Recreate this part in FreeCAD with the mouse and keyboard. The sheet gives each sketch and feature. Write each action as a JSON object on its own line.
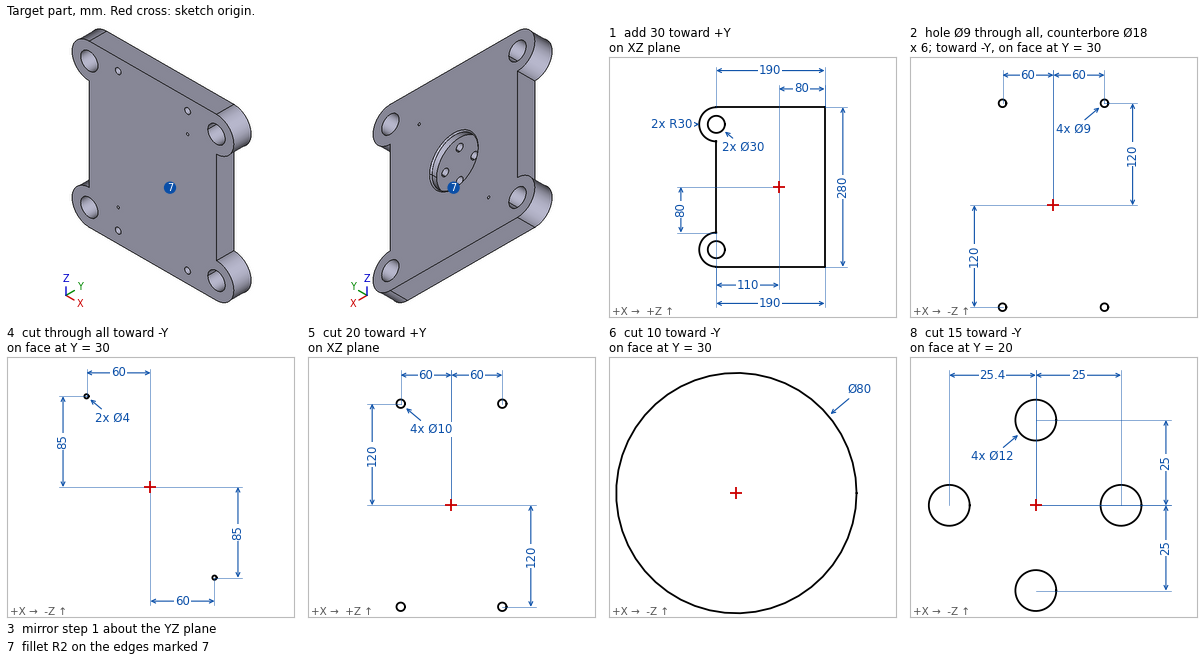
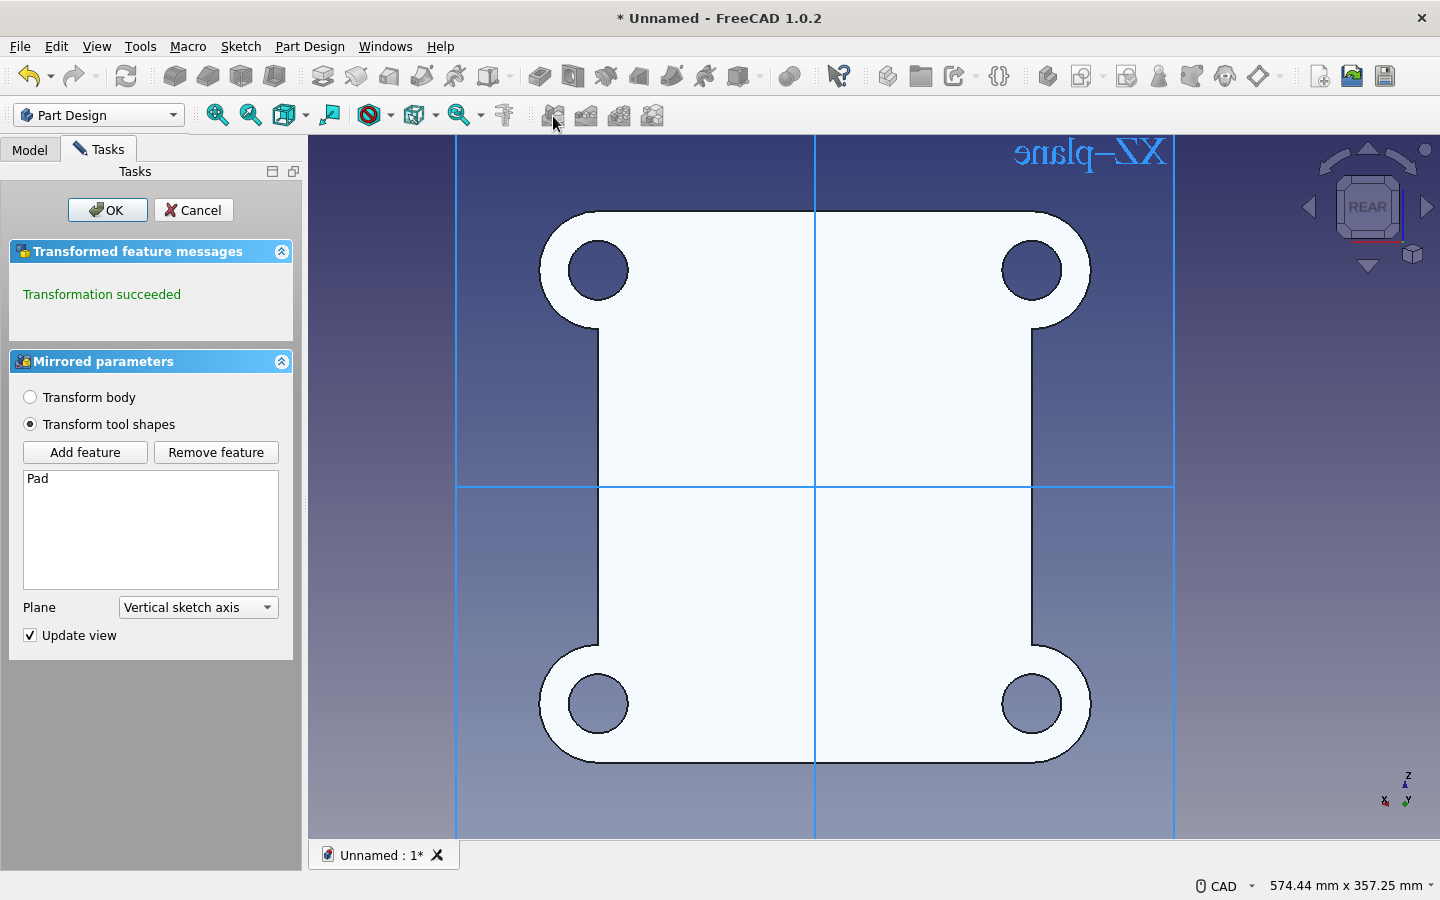
{"action": "left_click", "coordinate": [199, 608]}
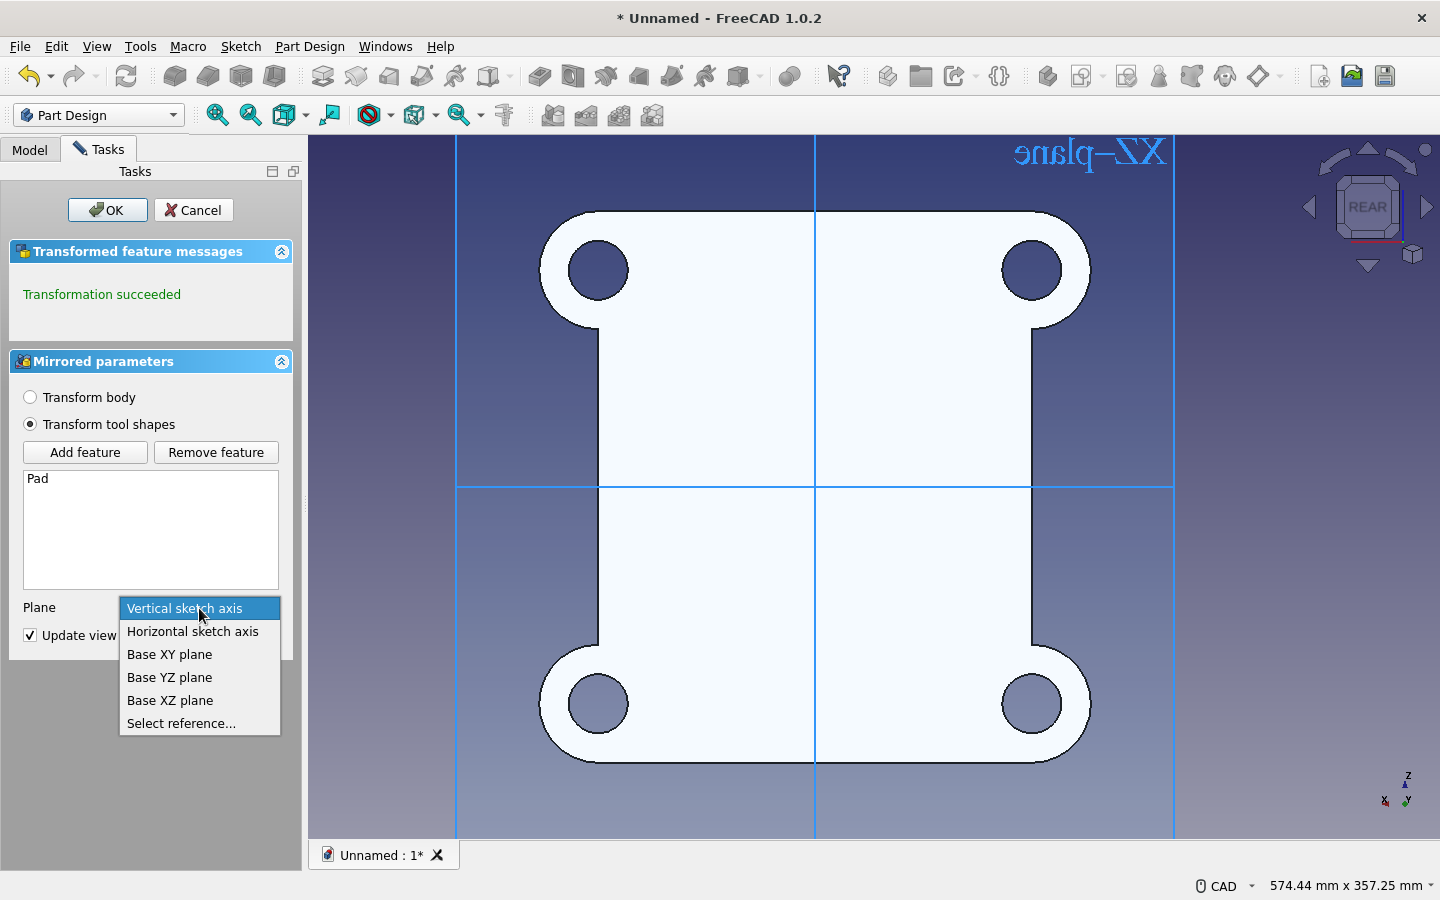
{"action": "left_click", "coordinate": [198, 678]}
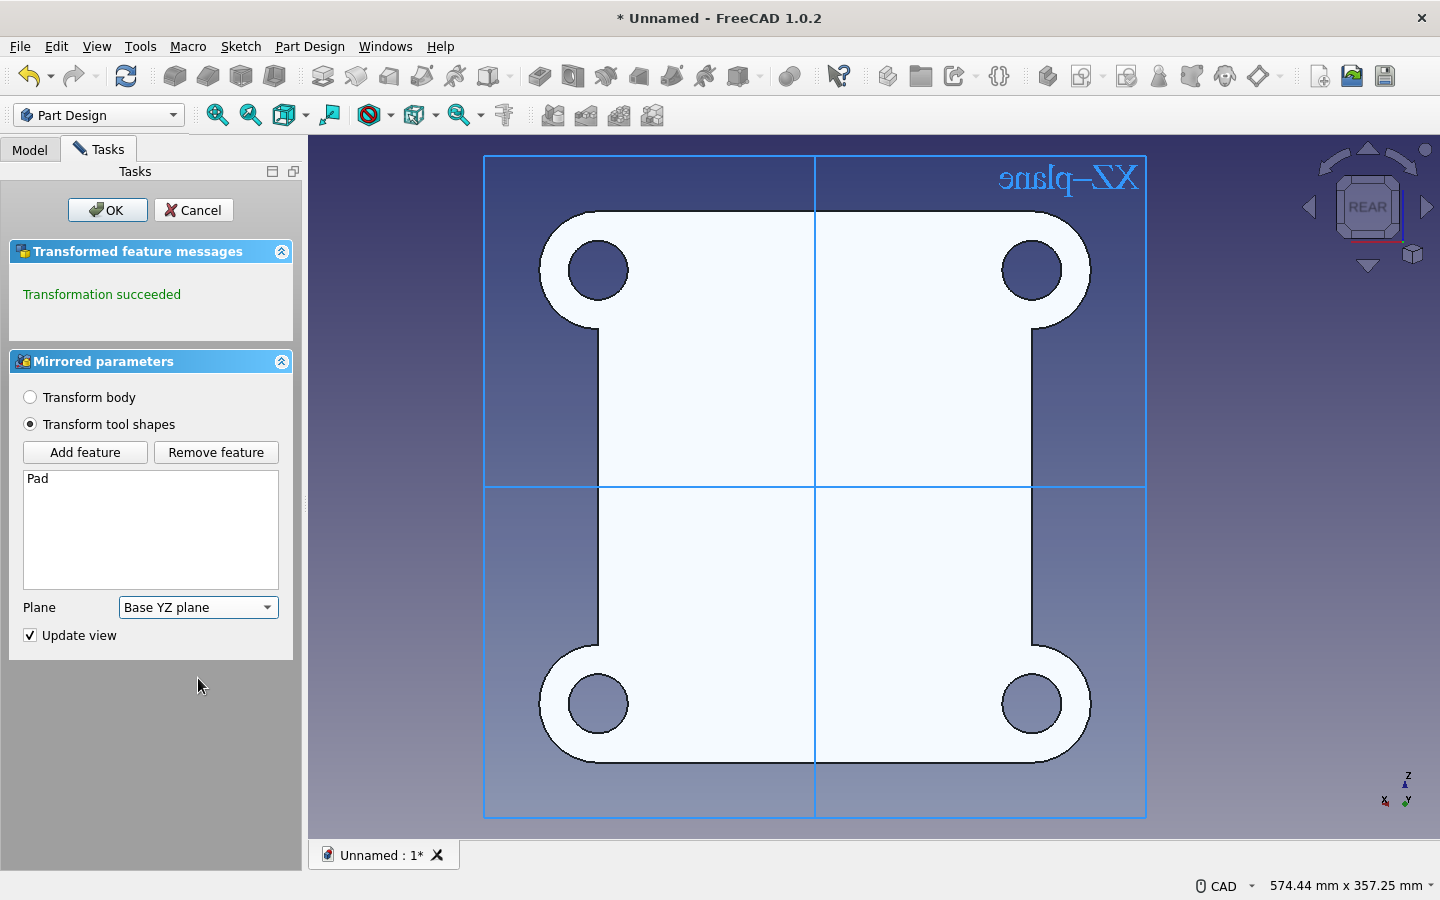
{"action": "left_click", "coordinate": [108, 210]}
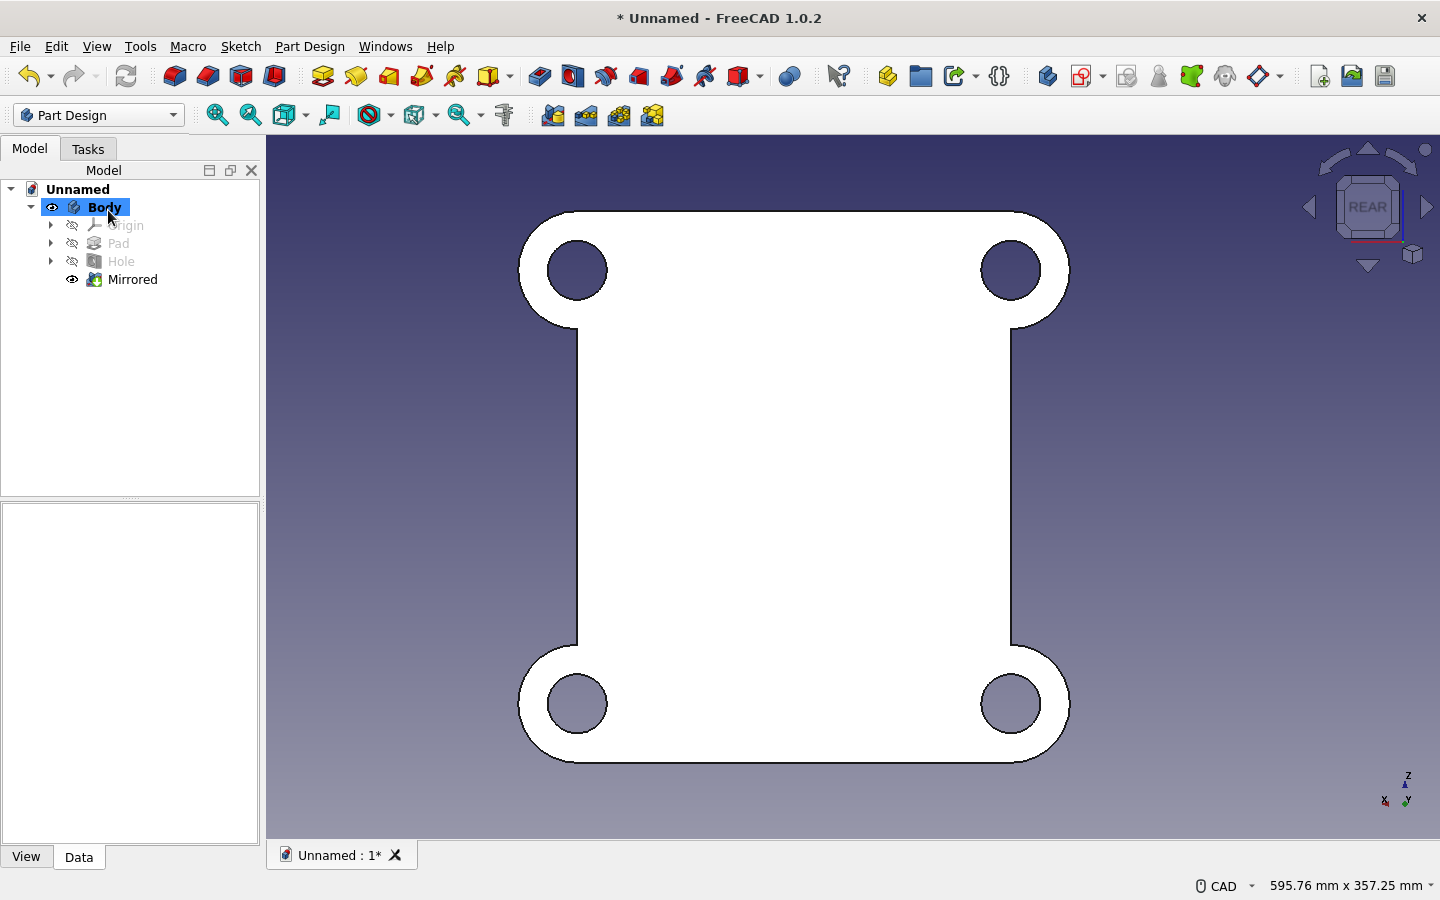
{"action": "left_click", "coordinate": [794, 486]}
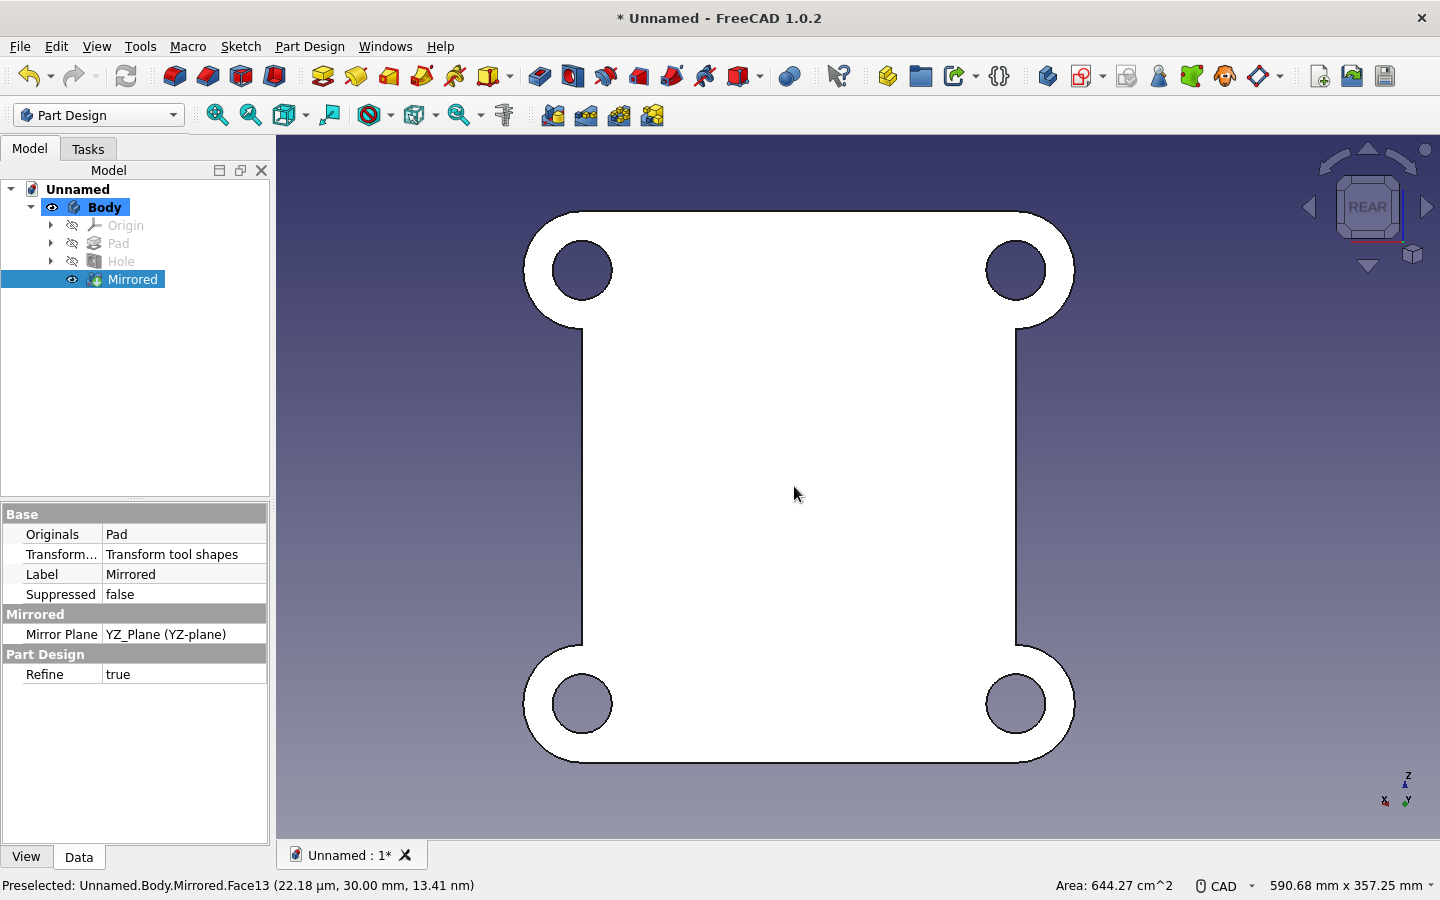
{"action": "left_click", "coordinate": [1080, 76]}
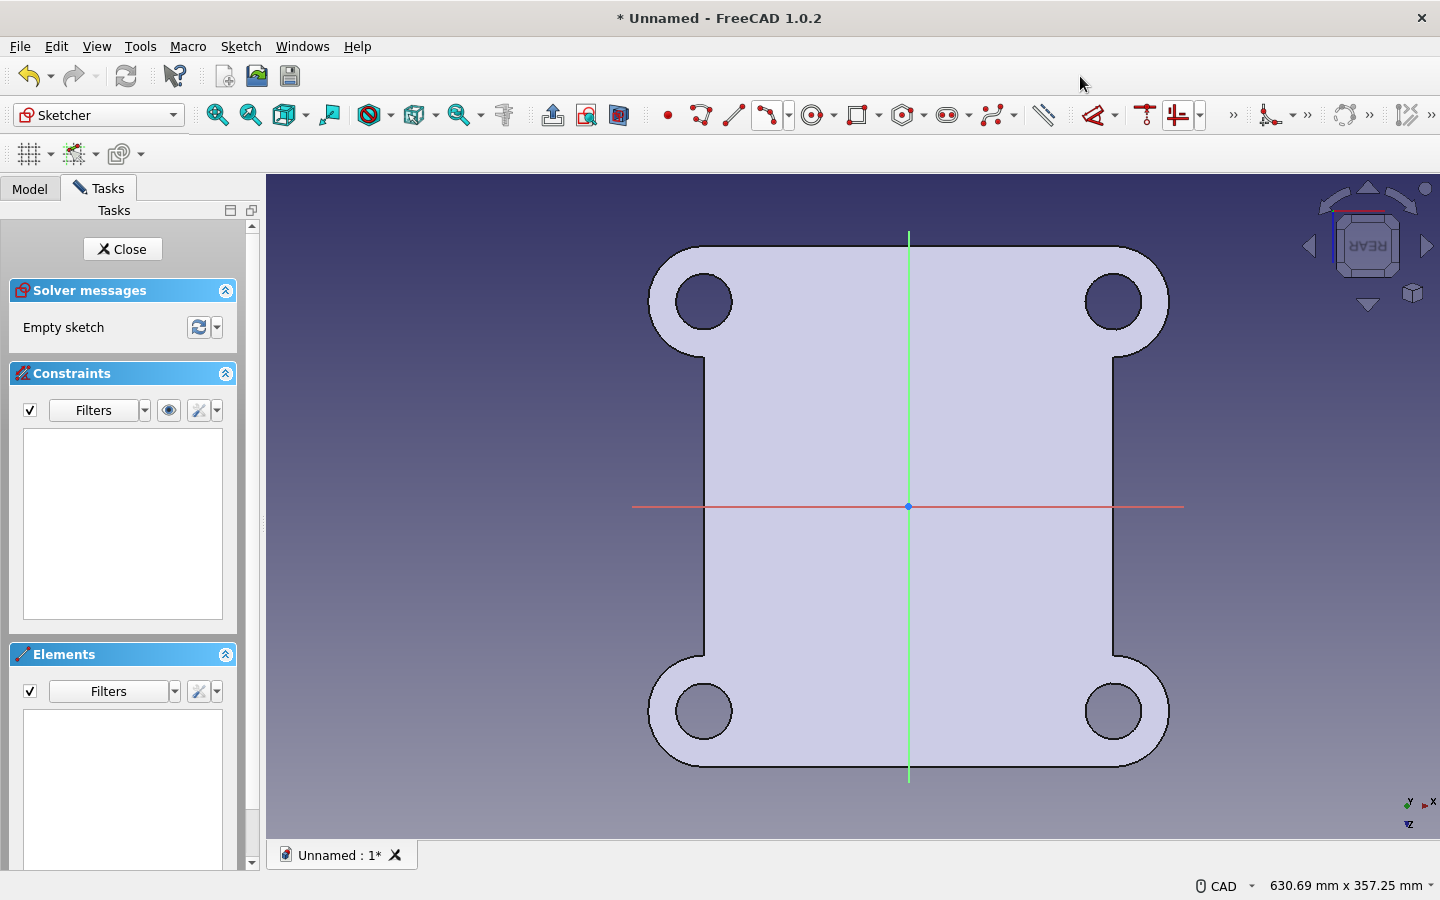
{"action": "left_click", "coordinate": [812, 116]}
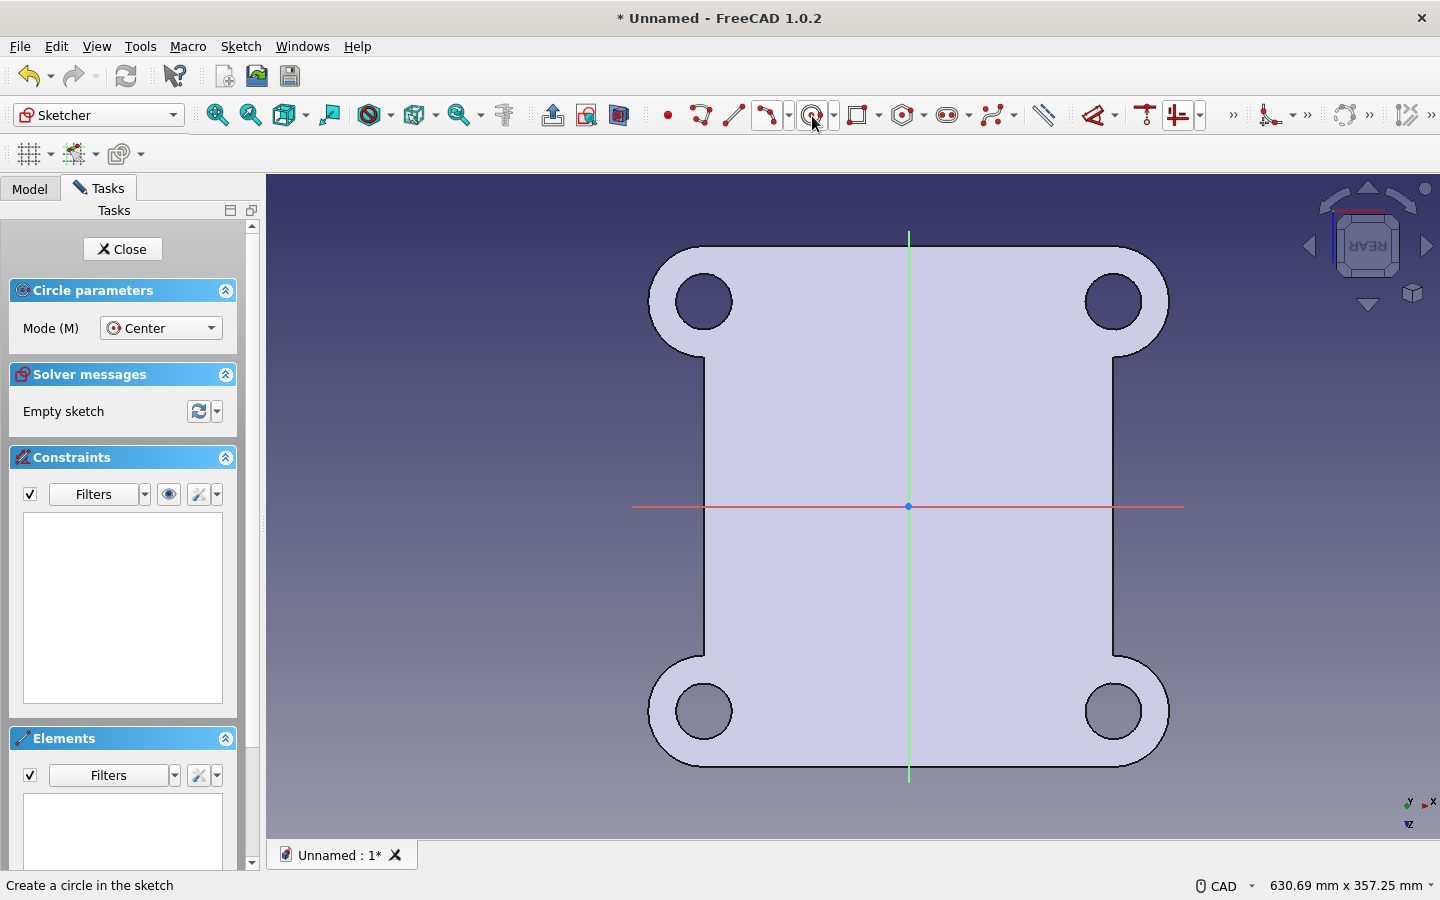
{"action": "scroll", "coordinate": [797, 348], "scroll_direction": "up", "scroll_amount": 10}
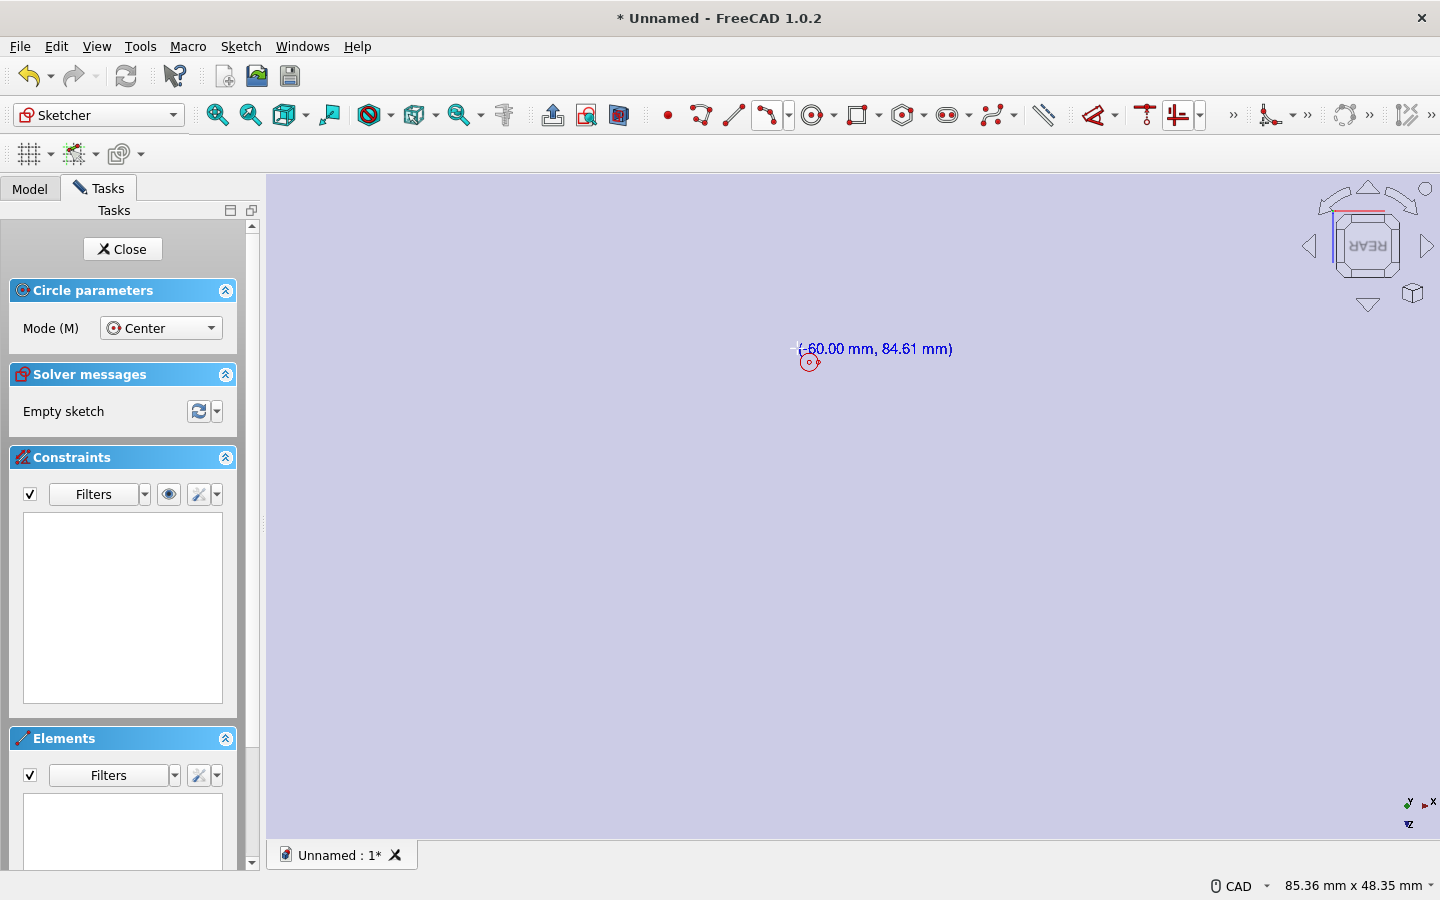
{"action": "scroll", "coordinate": [619, 306], "scroll_direction": "down", "scroll_amount": 9}